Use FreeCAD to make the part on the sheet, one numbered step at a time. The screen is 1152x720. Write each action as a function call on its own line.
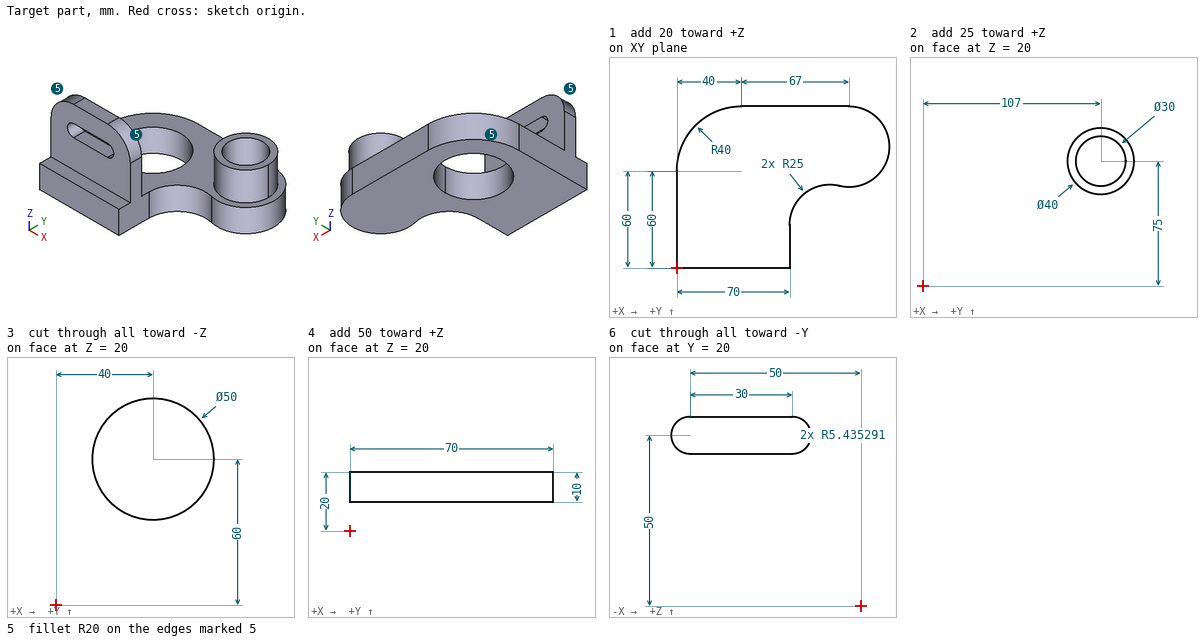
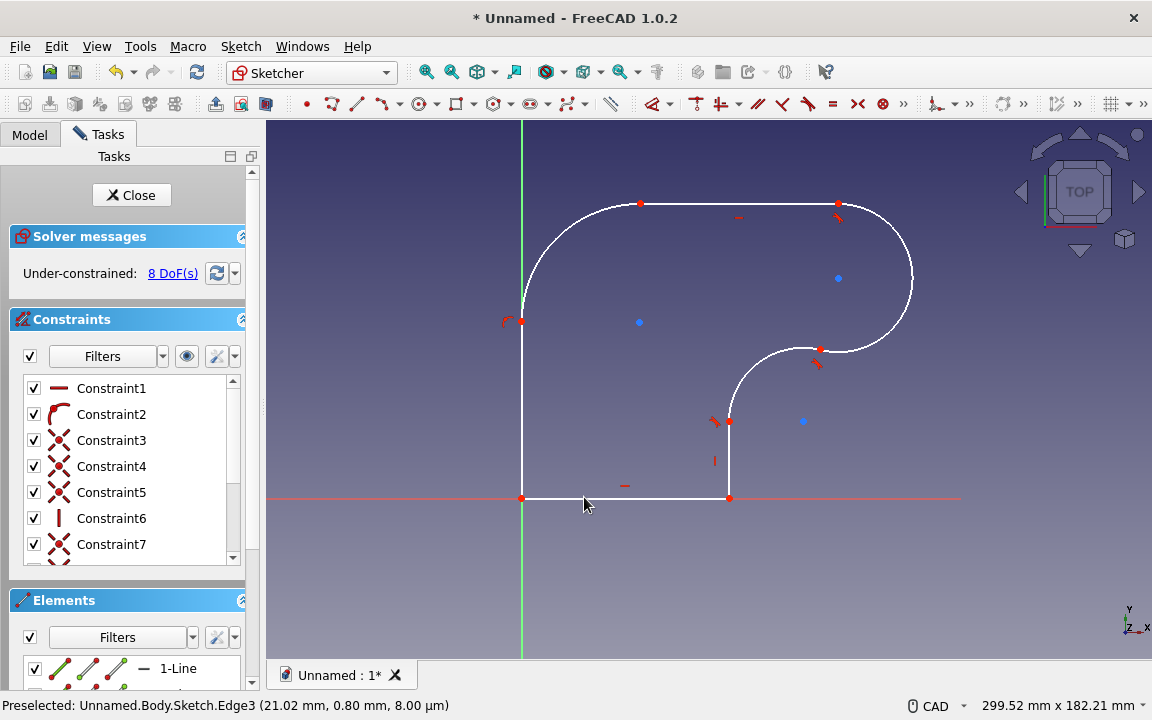
click(781, 351)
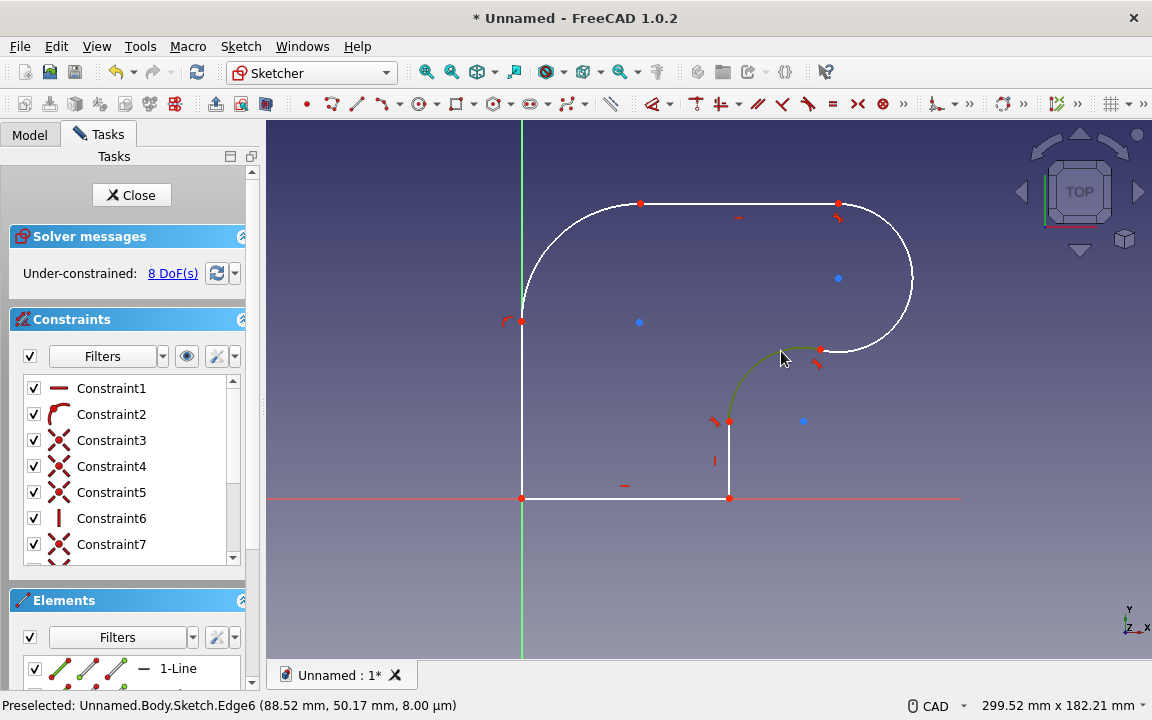
click(890, 331)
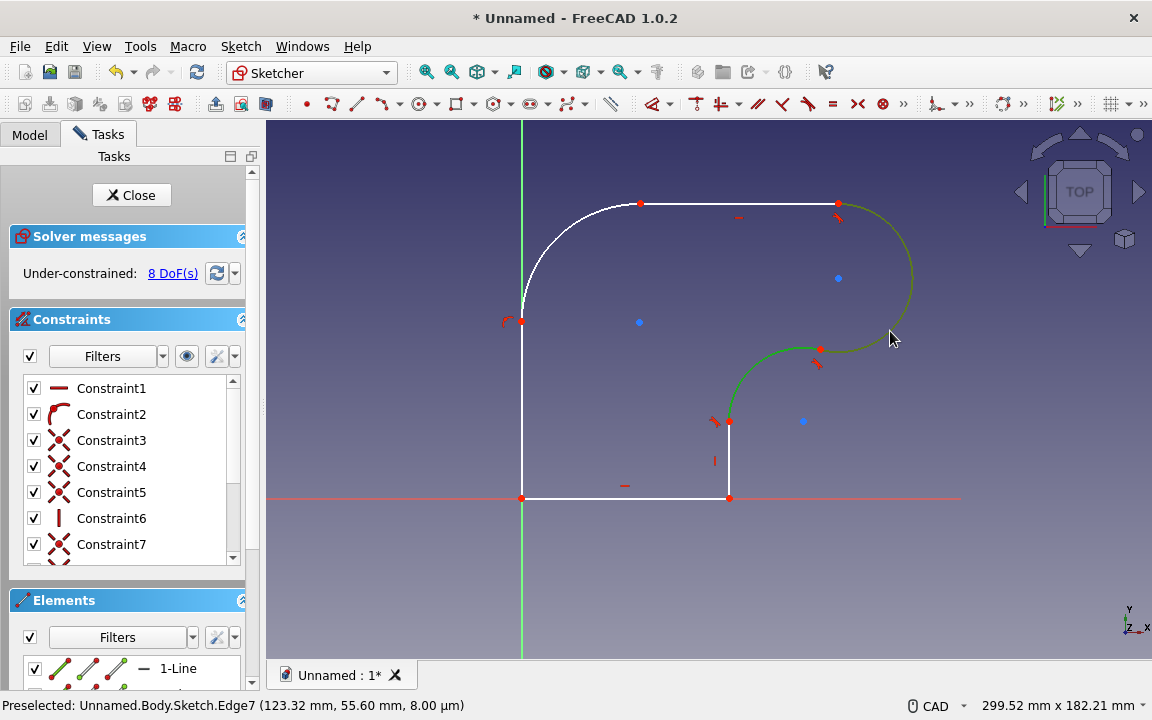
click(833, 104)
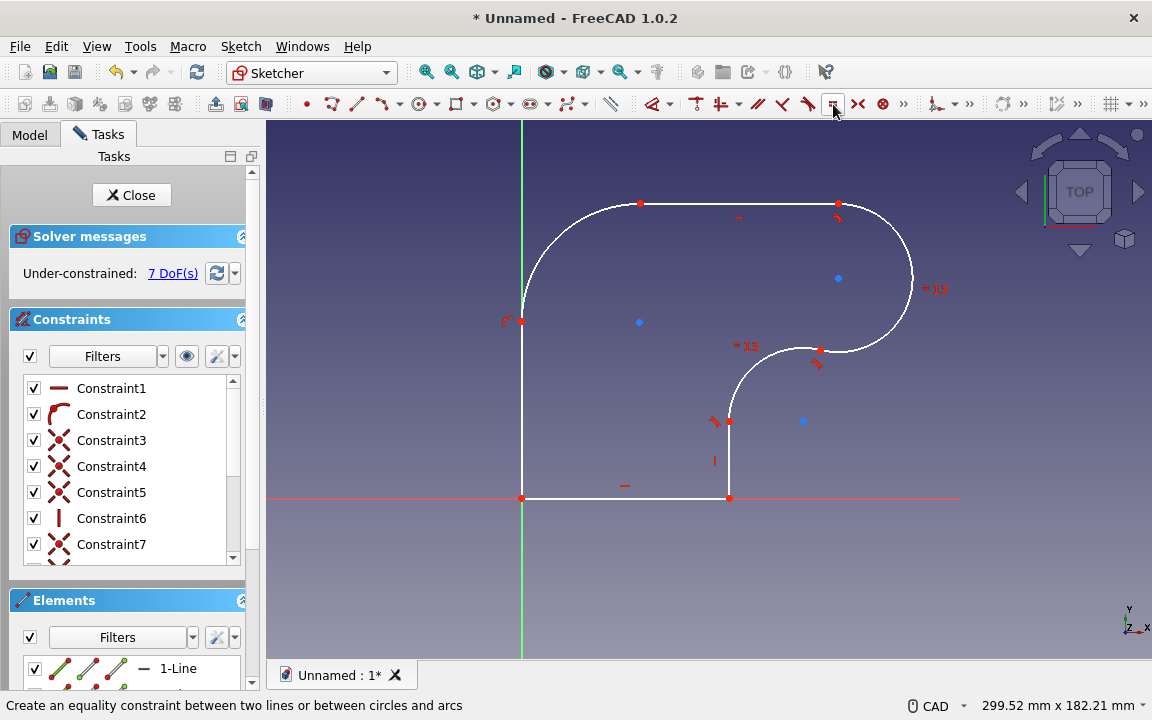
click(652, 104)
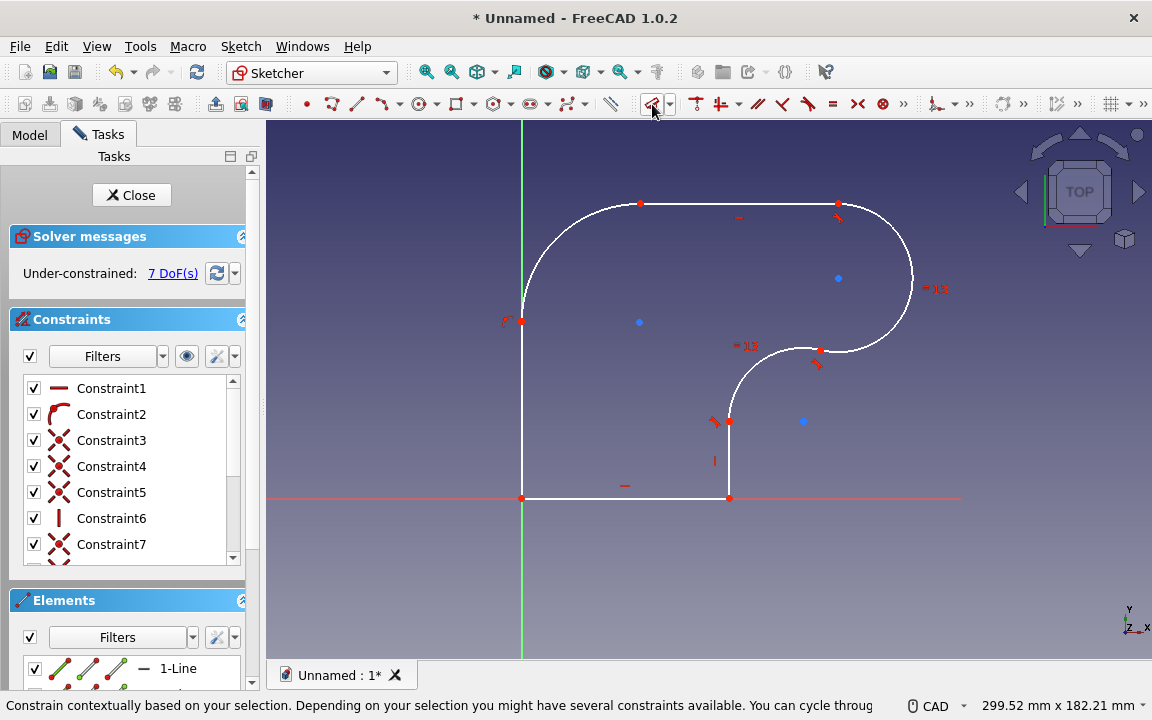
click(586, 217)
click(571, 189)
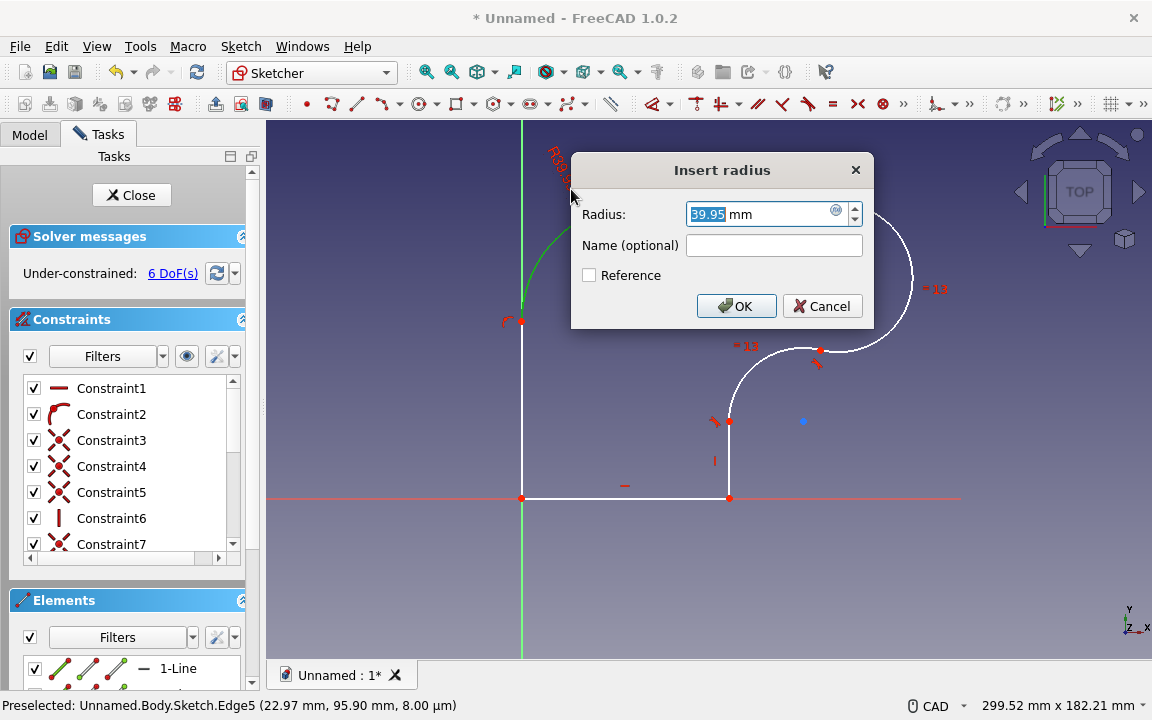
text(40)
key(Return)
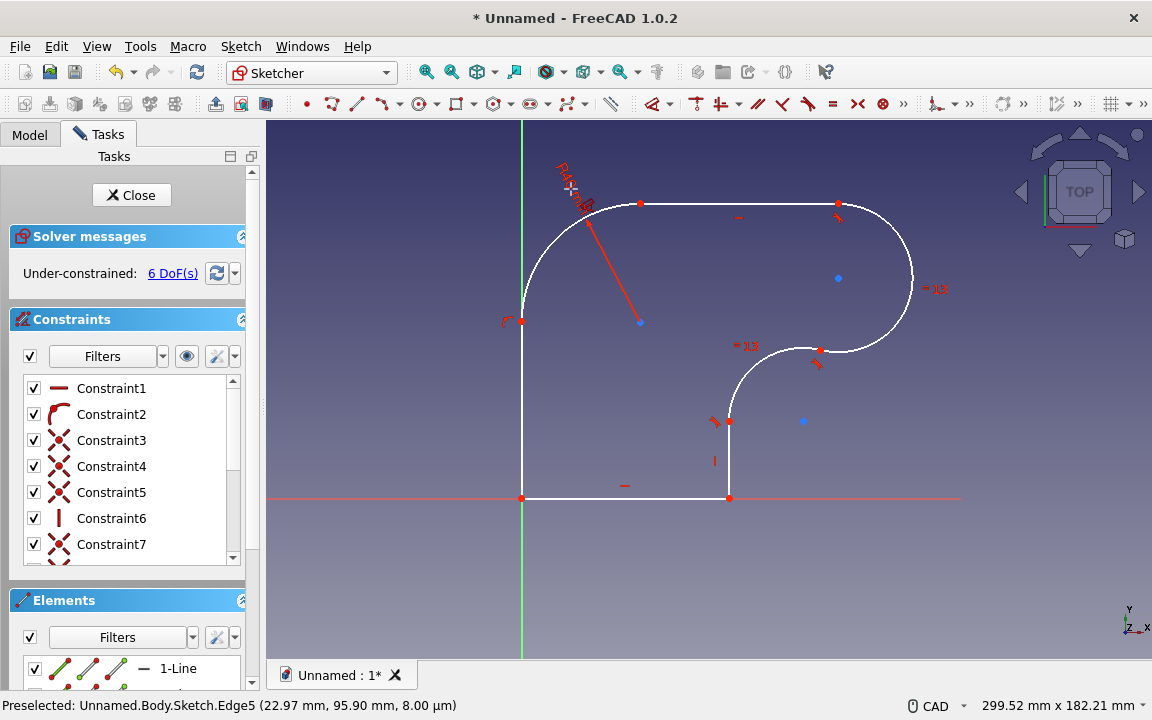
click(781, 351)
click(771, 320)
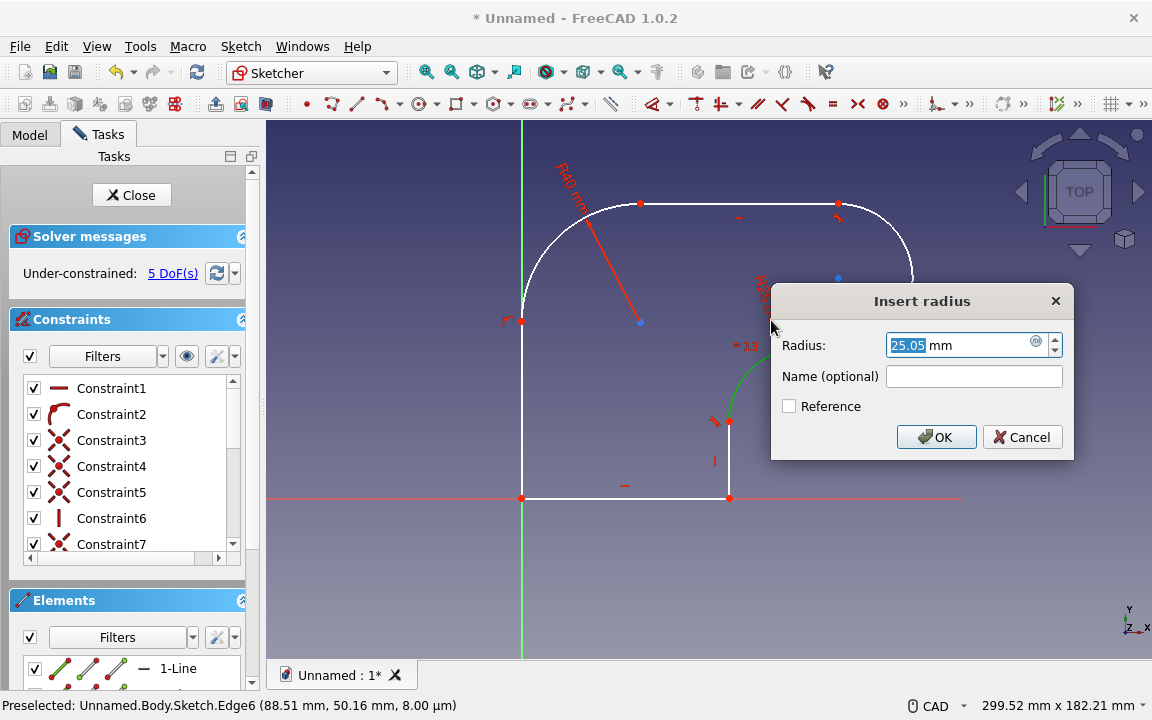
text(25)
key(Return)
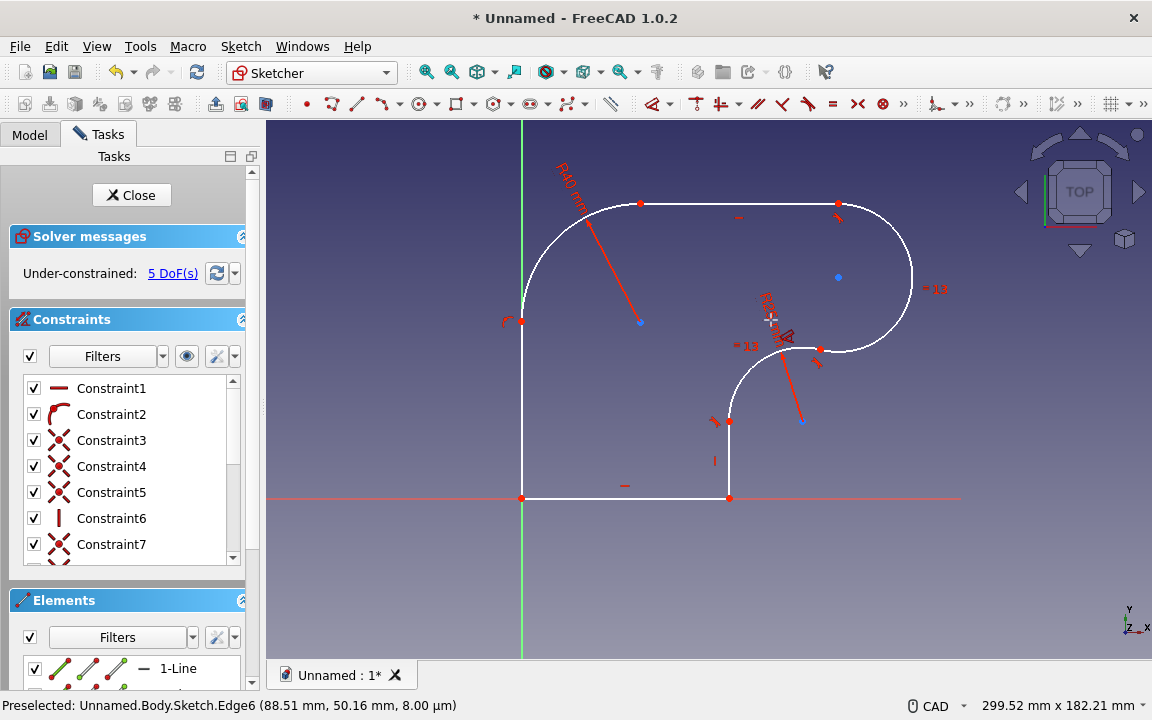
click(779, 204)
click(739, 170)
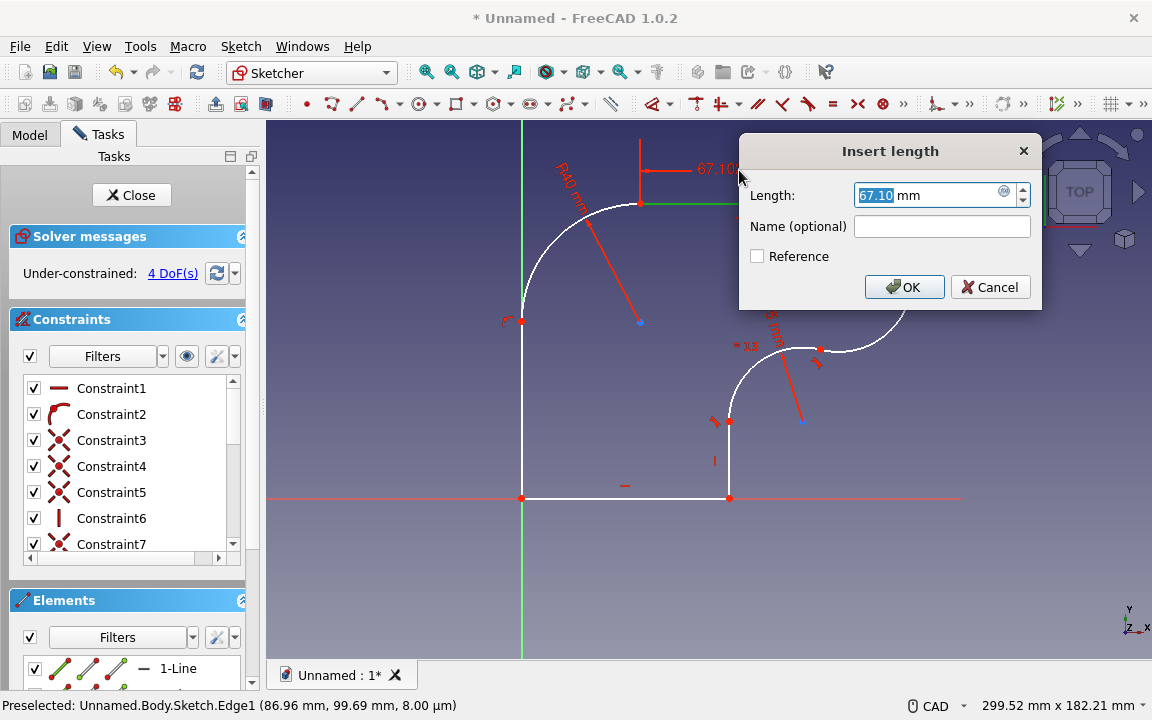
text(67)
key(Return)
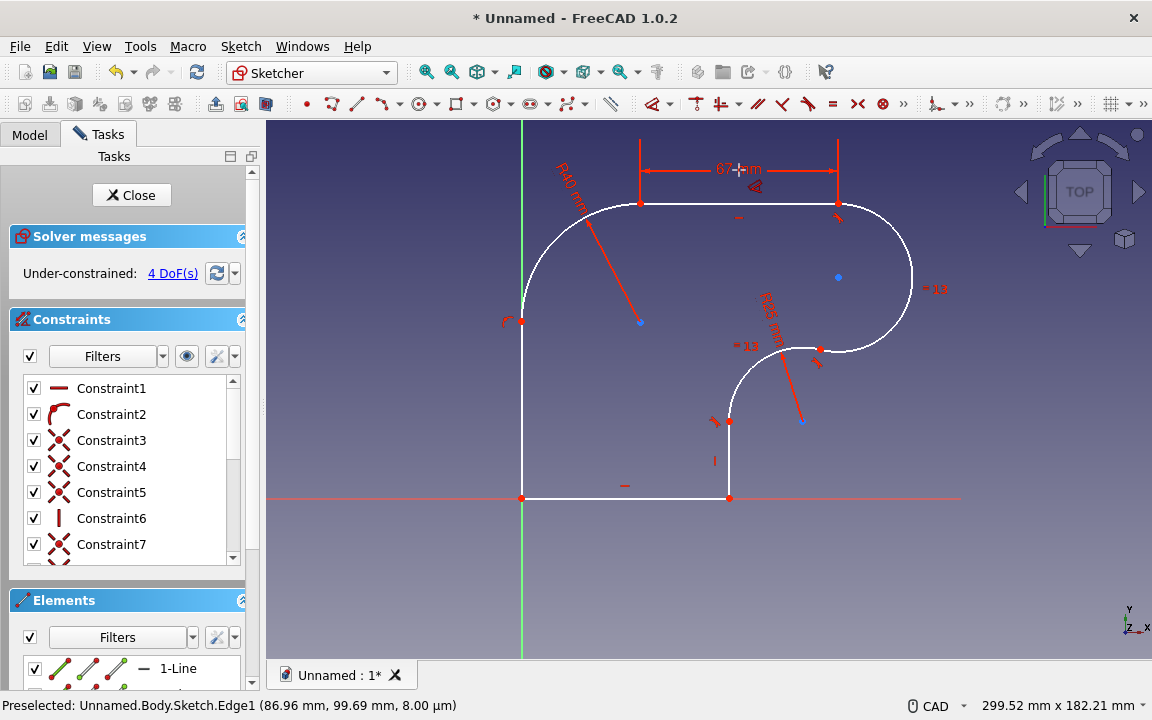
click(522, 375)
click(488, 410)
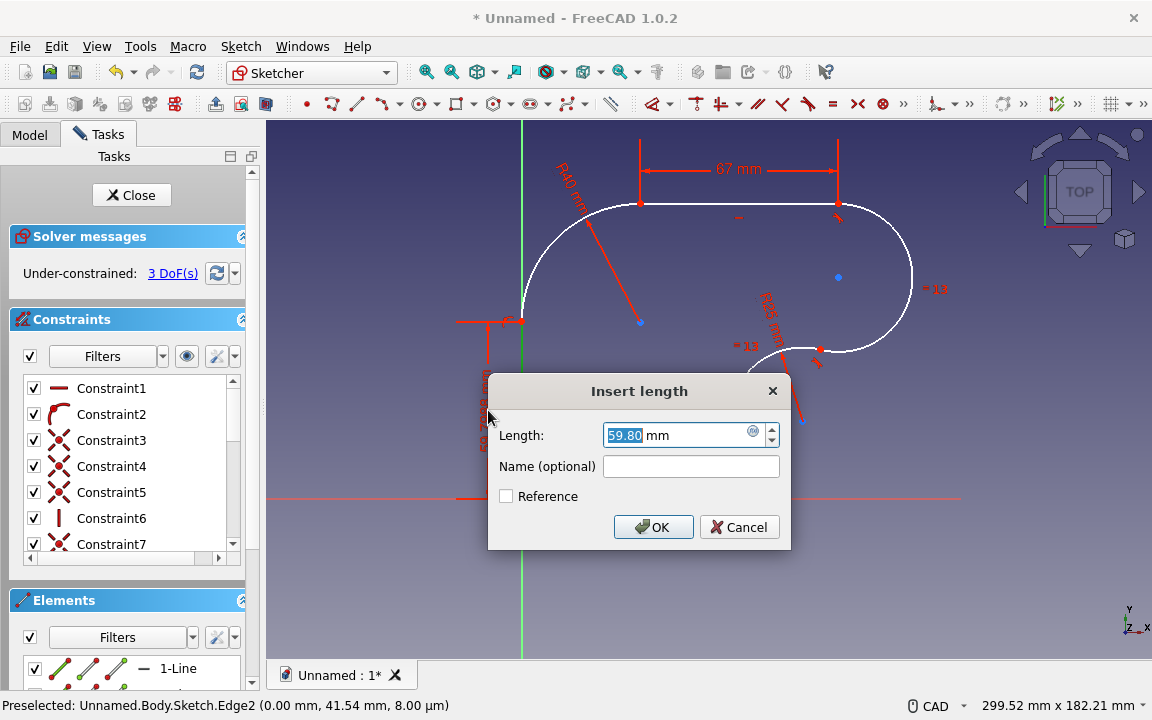
text(60)
key(Return)